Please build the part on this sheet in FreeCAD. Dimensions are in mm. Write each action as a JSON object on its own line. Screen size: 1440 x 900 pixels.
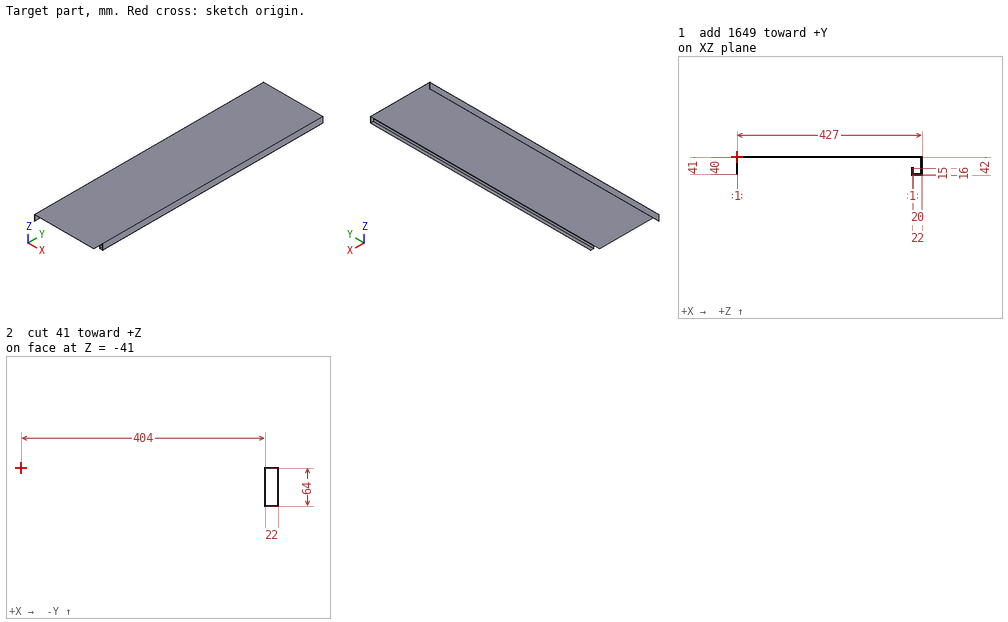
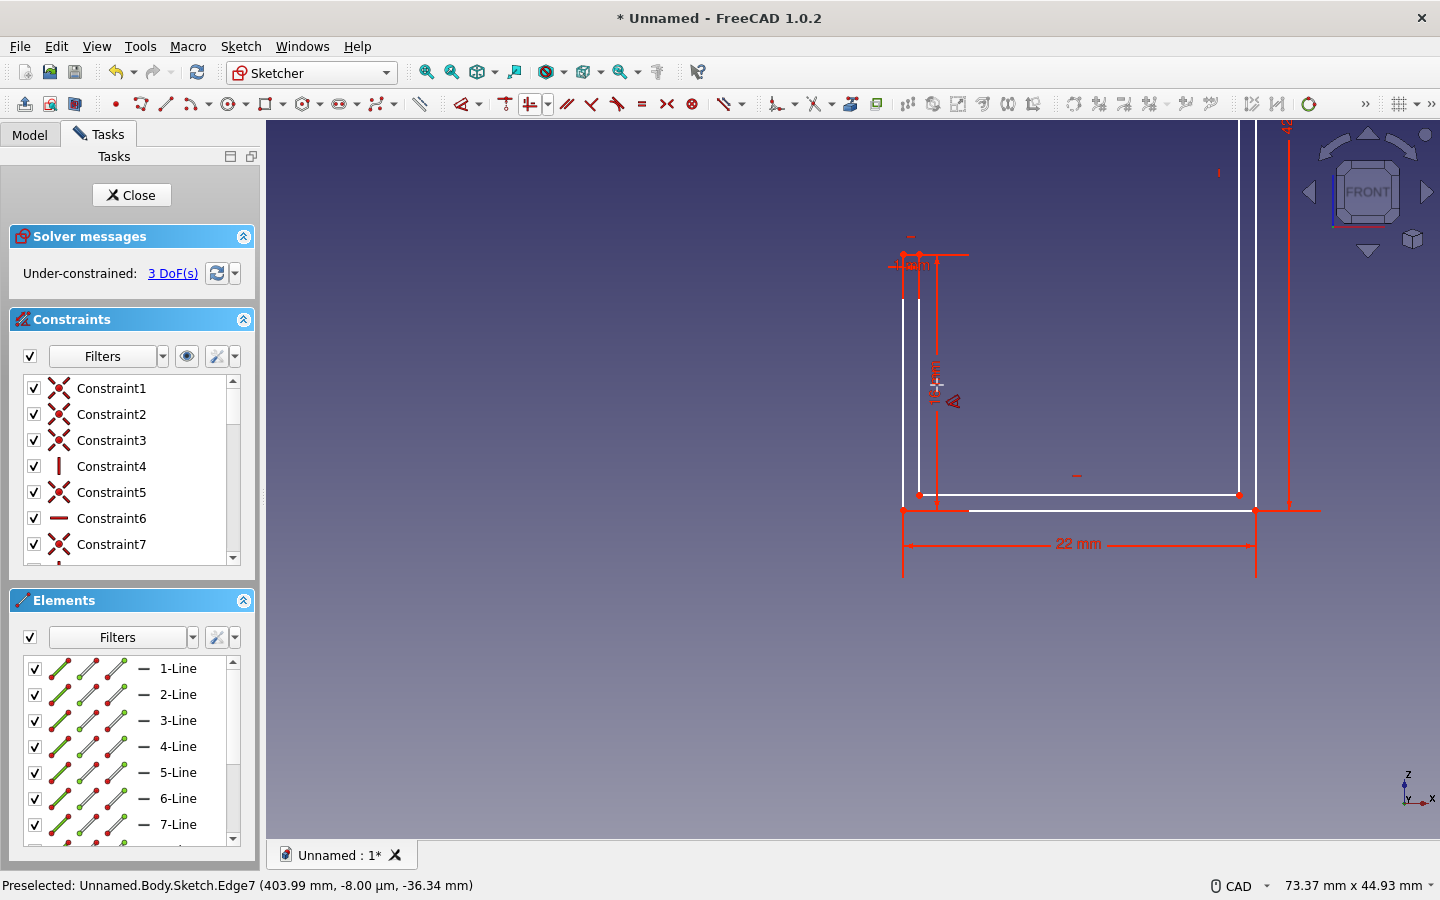
{"action": "left_click", "coordinate": [919, 327]}
{"action": "left_click", "coordinate": [953, 320]}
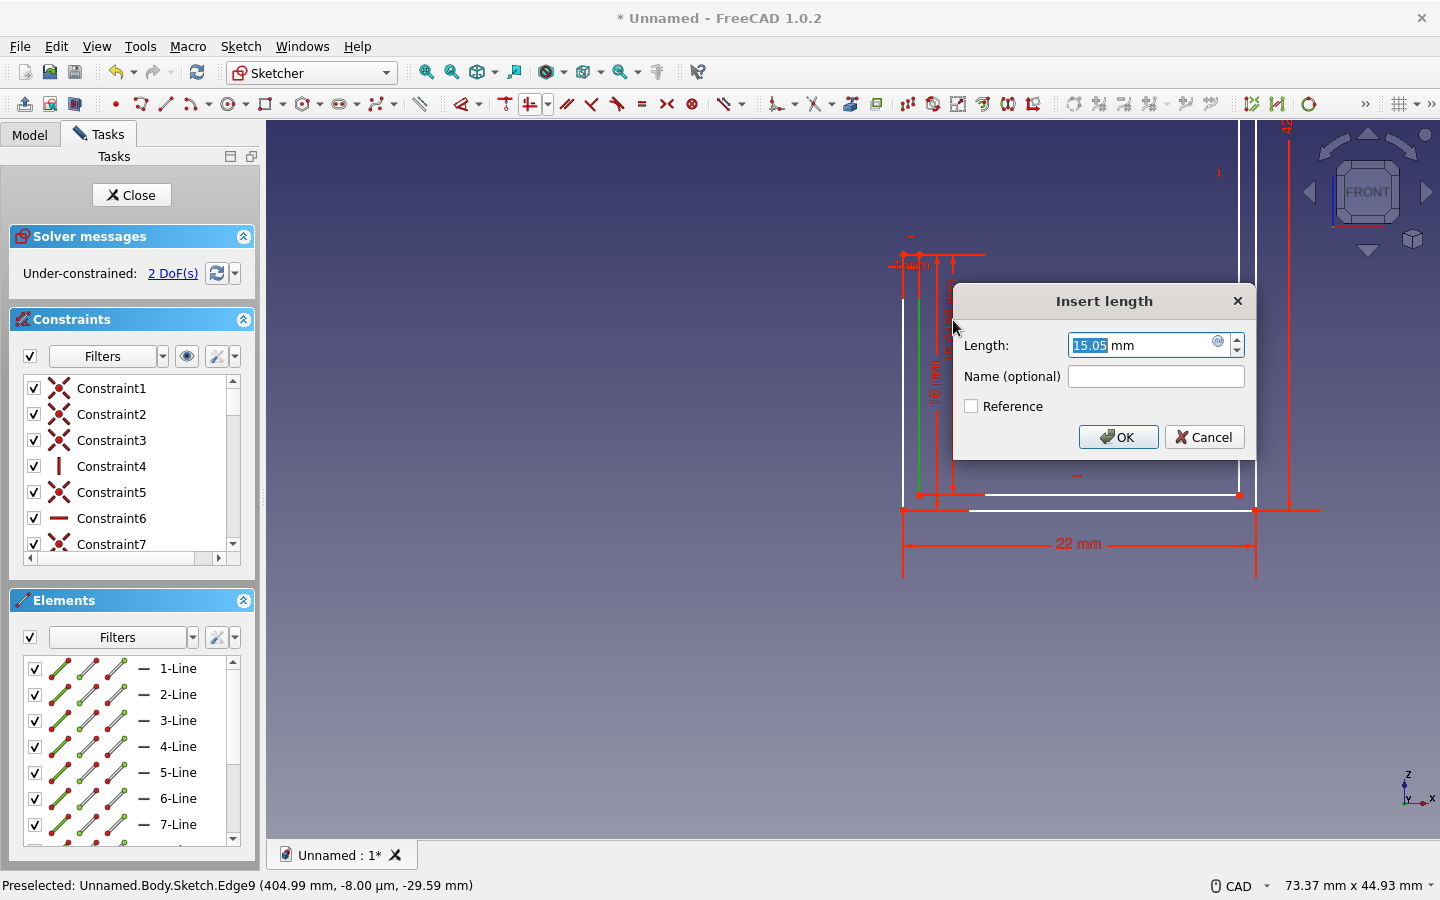
{"action": "type", "text": "15"}
{"action": "key", "text": "Return"}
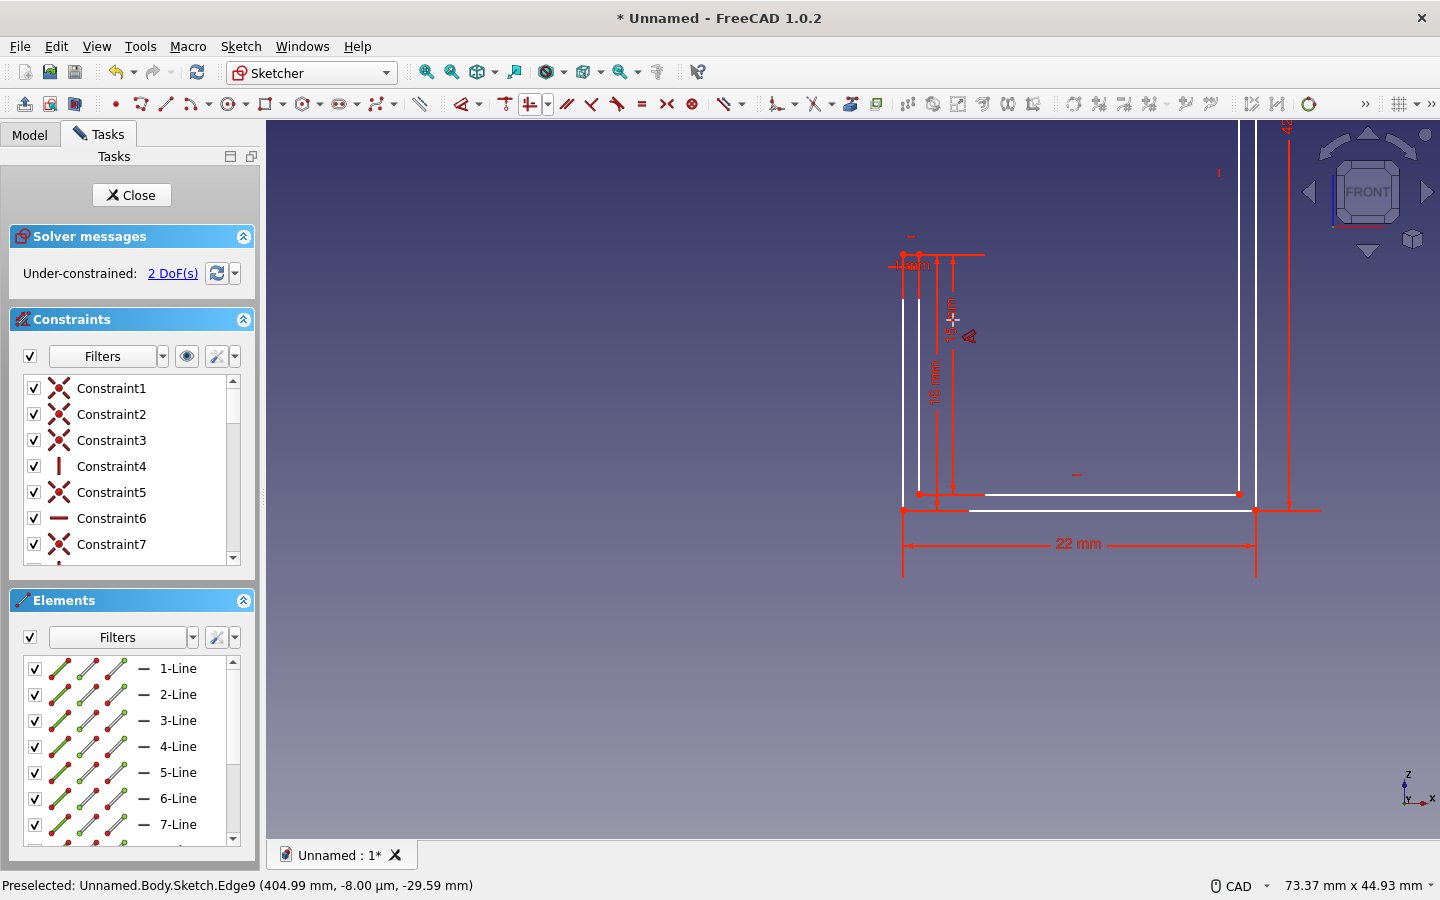
{"action": "left_click", "coordinate": [1015, 495]}
{"action": "left_click", "coordinate": [1006, 529]}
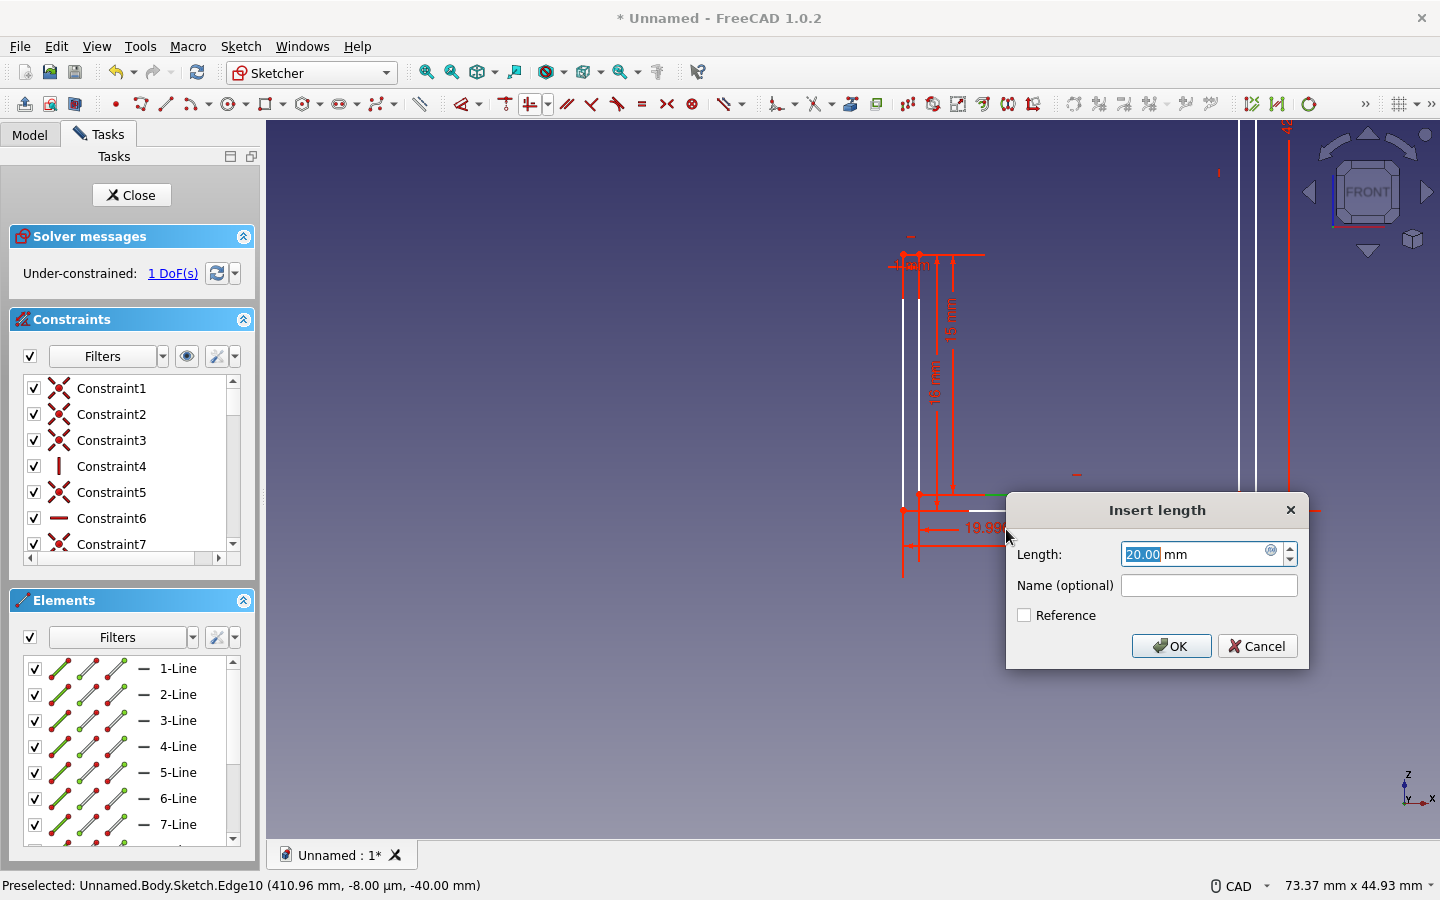
{"action": "type", "text": "20"}
{"action": "key", "text": "Return"}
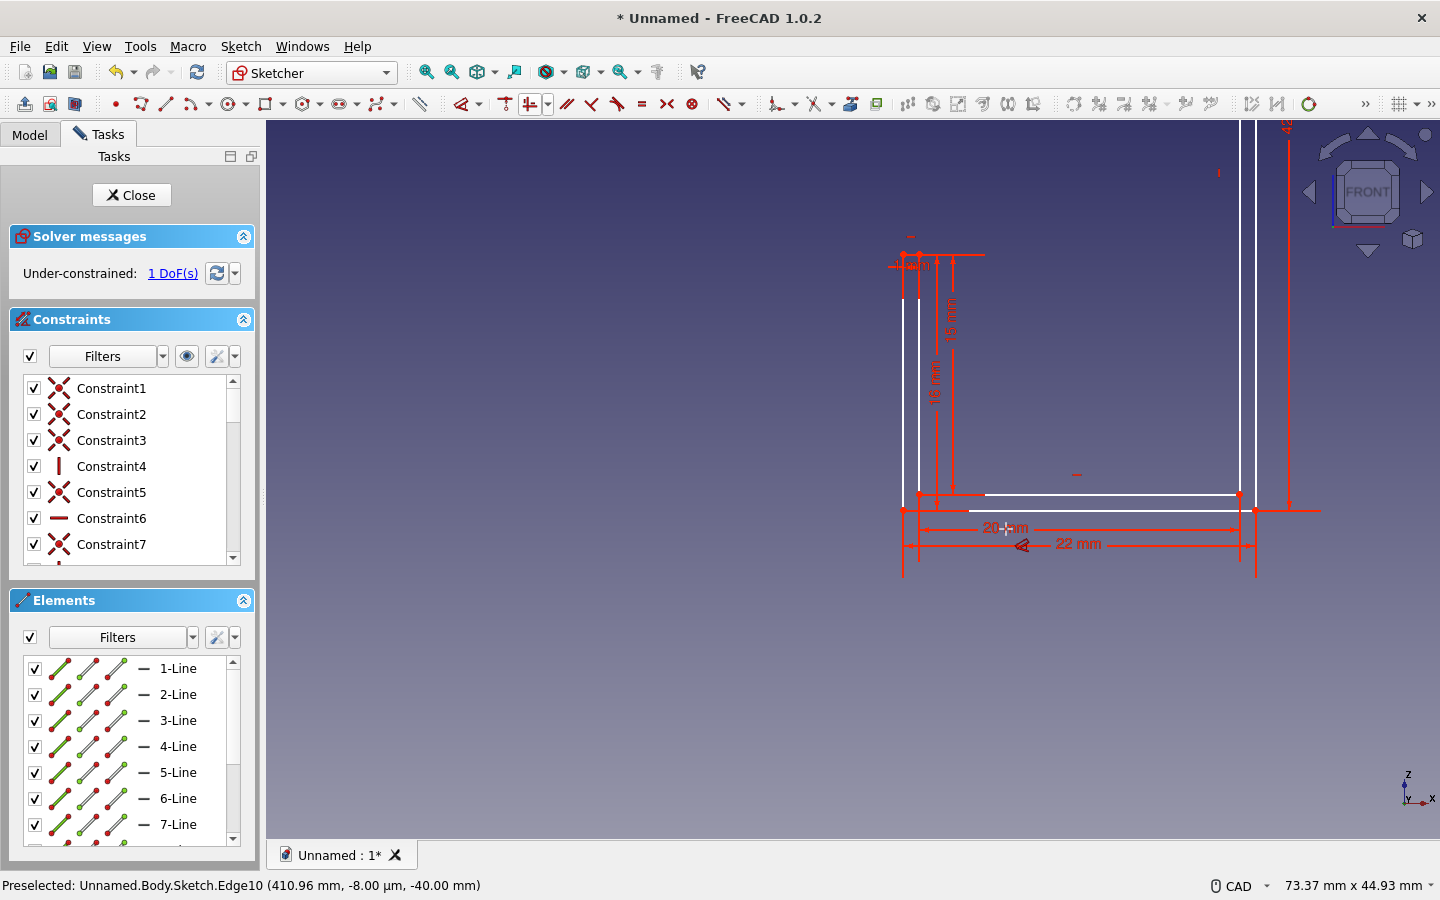
{"action": "scroll", "coordinate": [1151, 518], "scroll_direction": "down", "scroll_amount": 11}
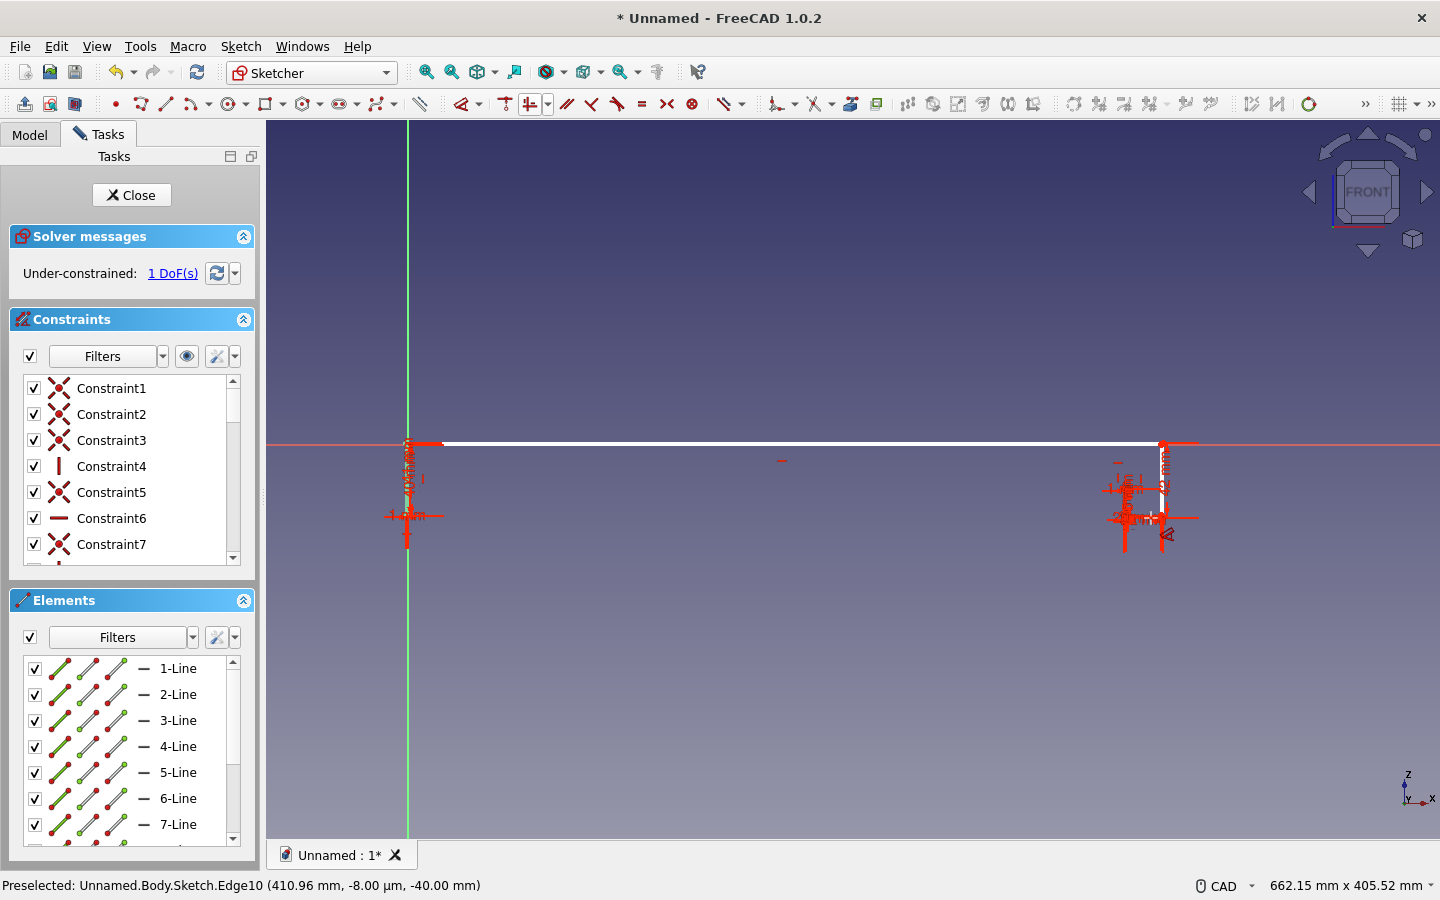
{"action": "scroll", "coordinate": [633, 443], "scroll_direction": "up", "scroll_amount": 11}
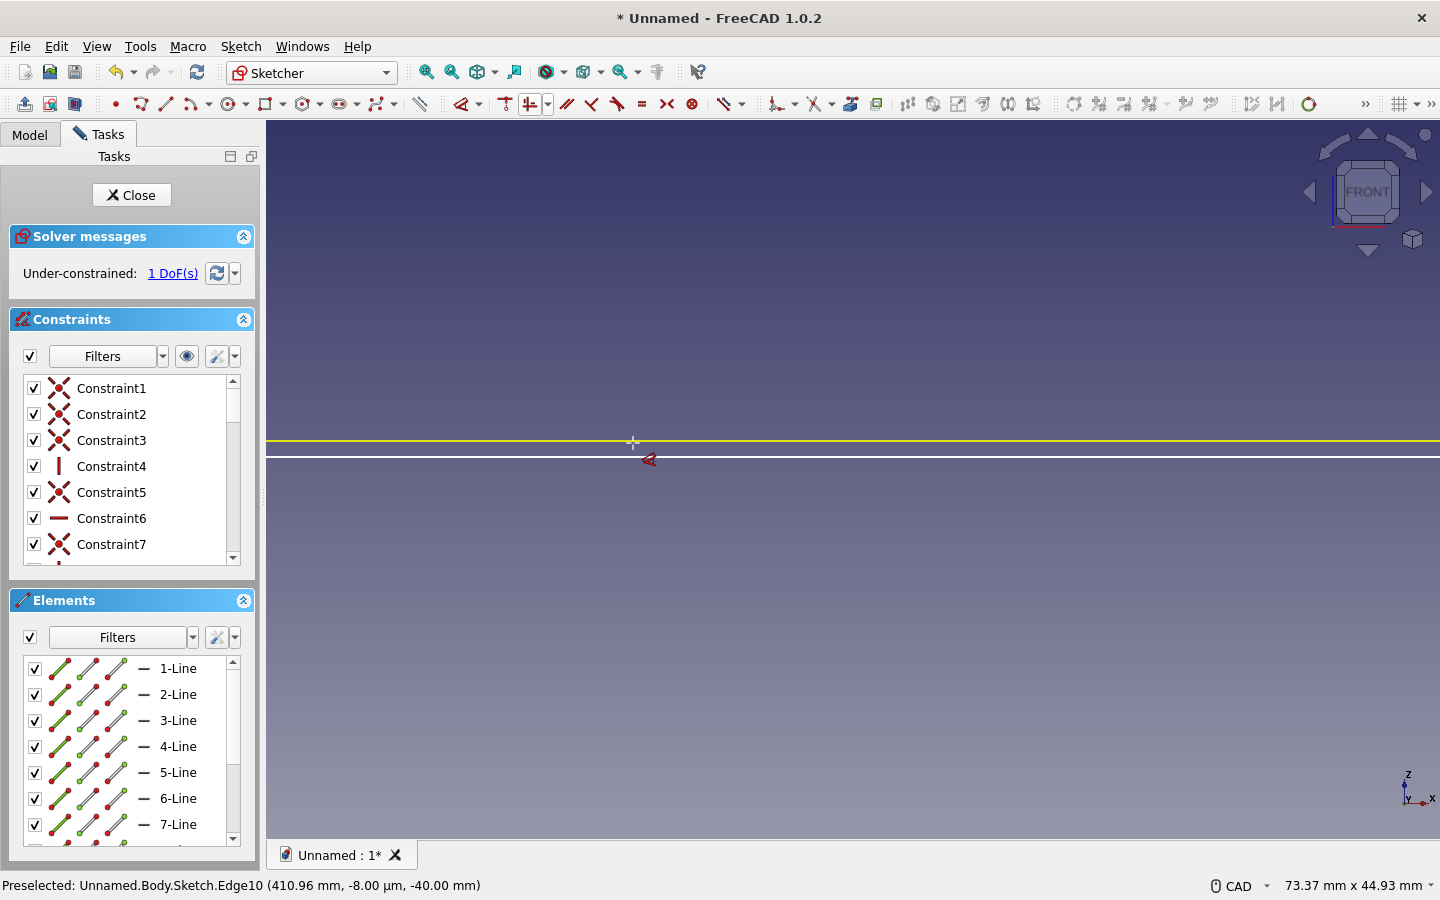
{"action": "left_click", "coordinate": [633, 441]}
{"action": "left_click", "coordinate": [784, 407]}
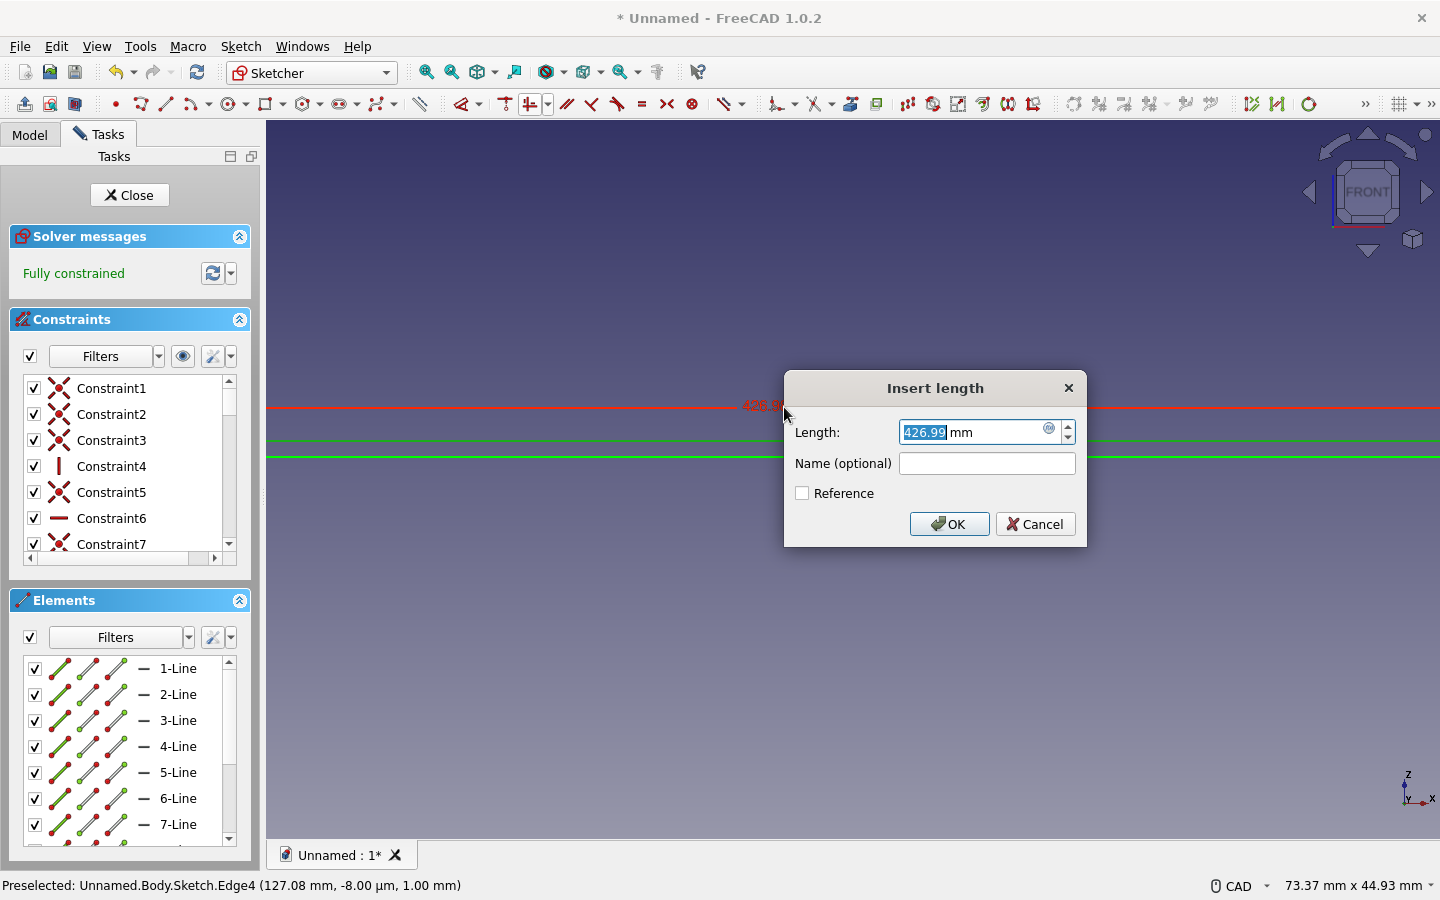
{"action": "type", "text": "427"}
{"action": "key", "text": "Return"}
{"action": "key", "text": "Escape"}